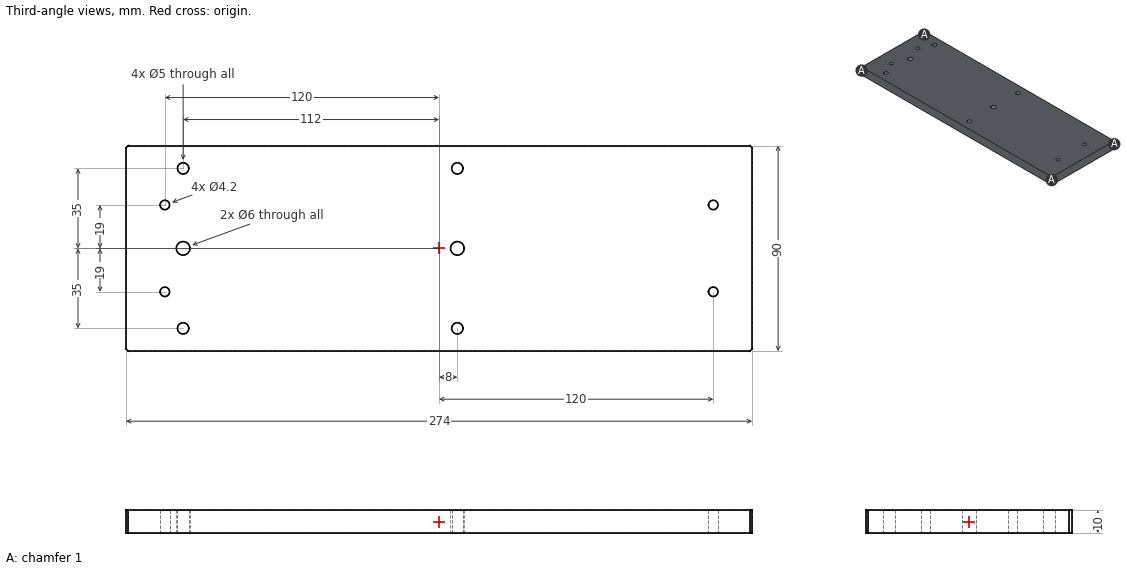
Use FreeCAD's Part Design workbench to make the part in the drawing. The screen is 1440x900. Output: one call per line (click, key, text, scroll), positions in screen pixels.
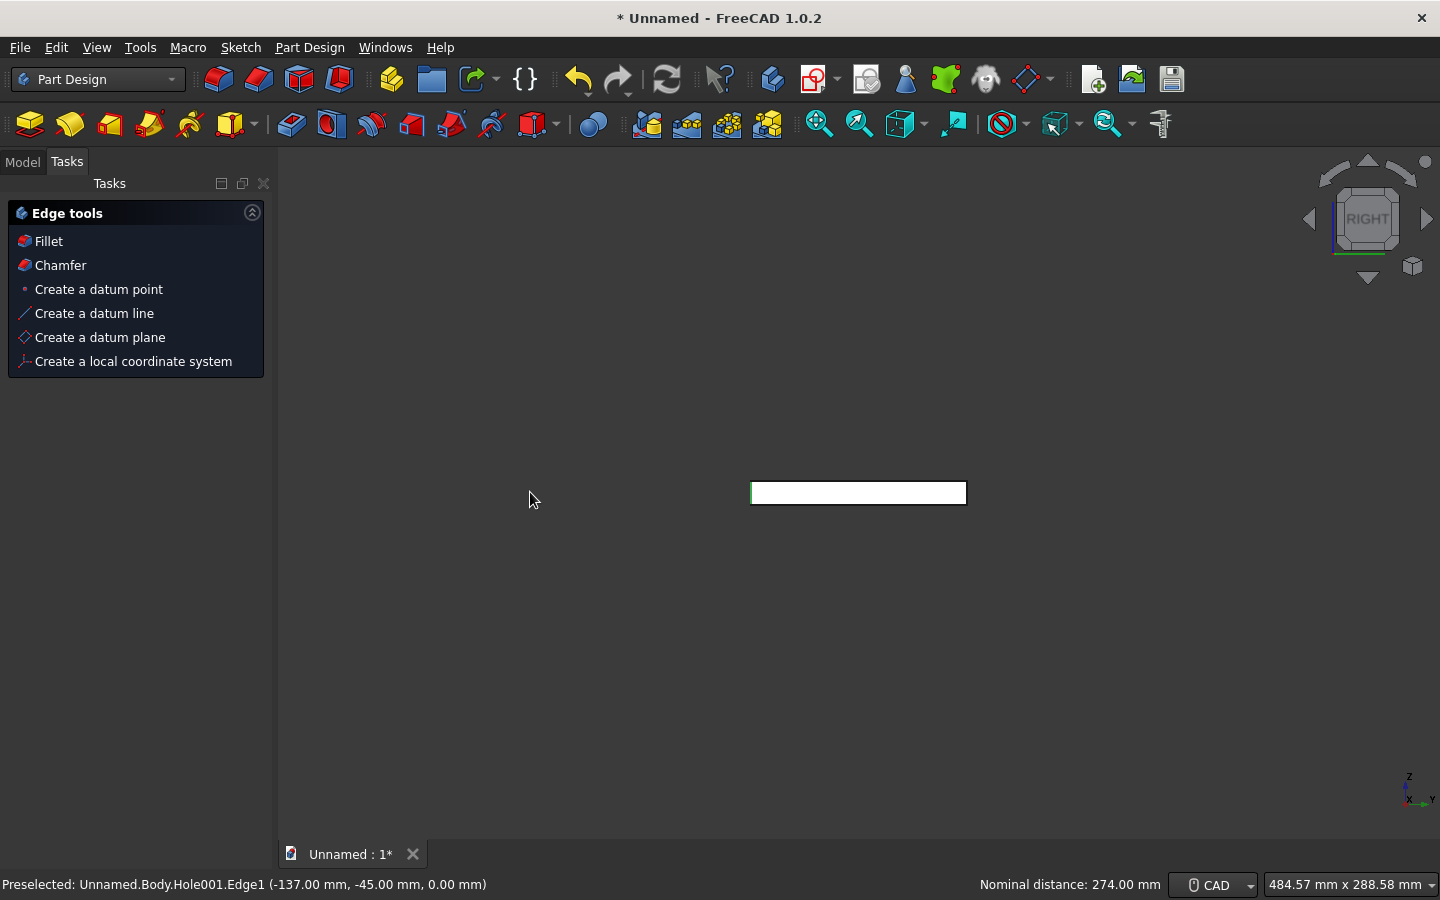
click(967, 492, ctrl)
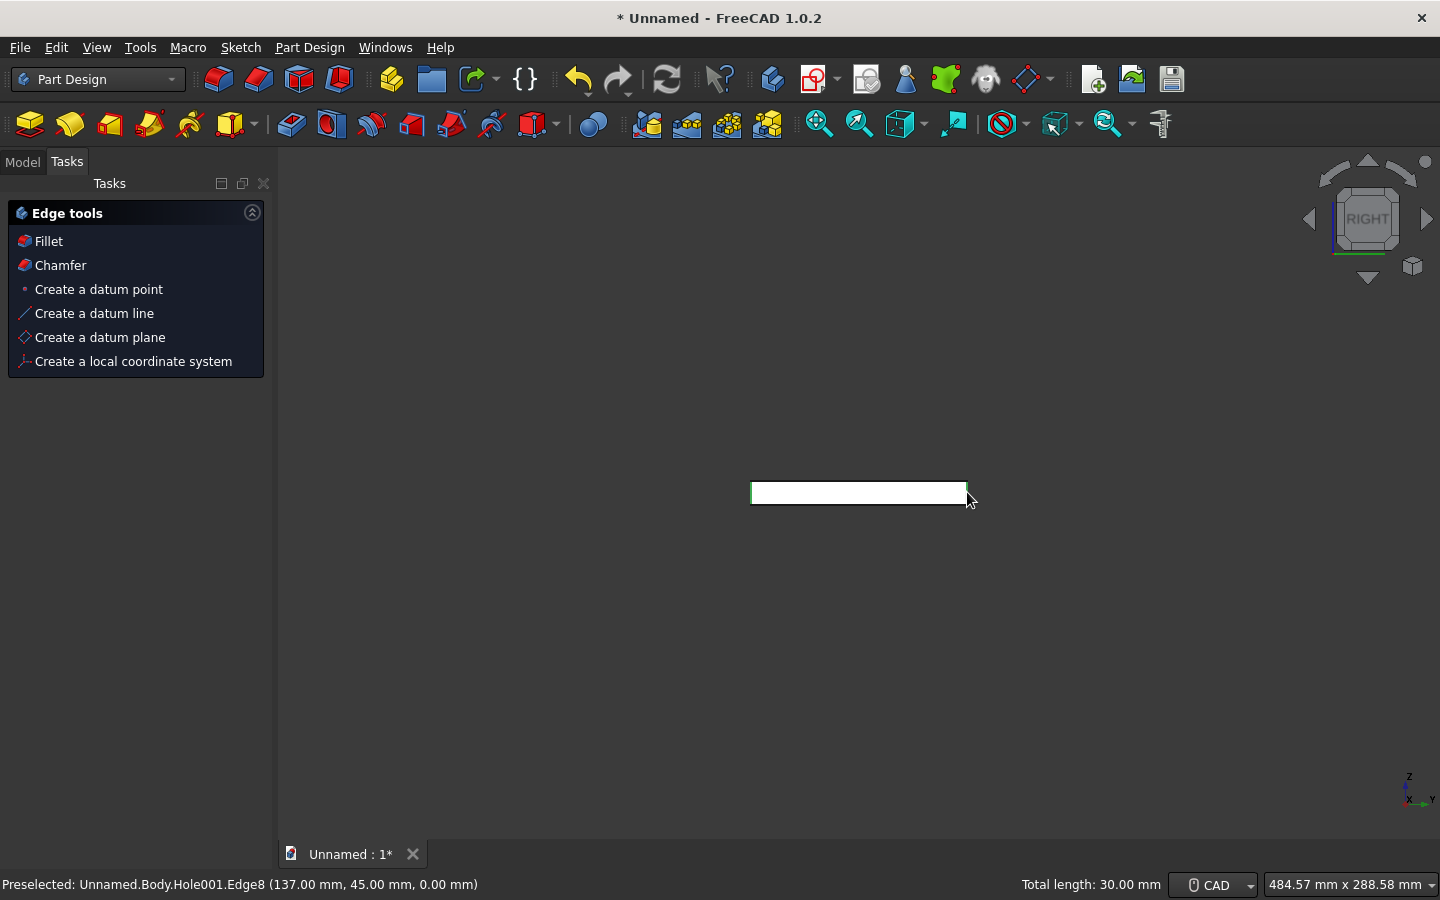
key(5)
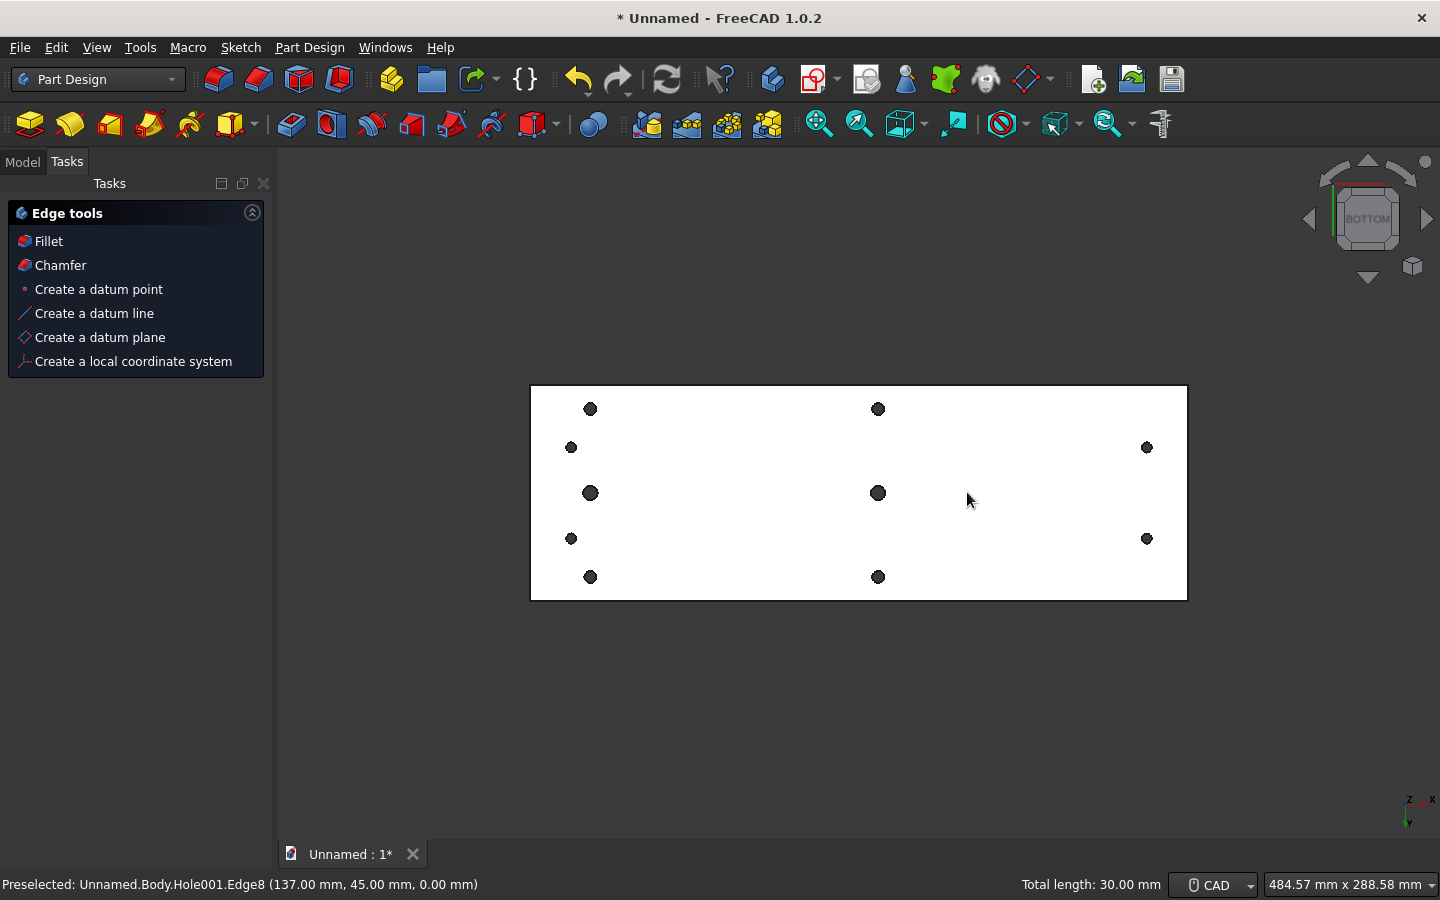
key(4)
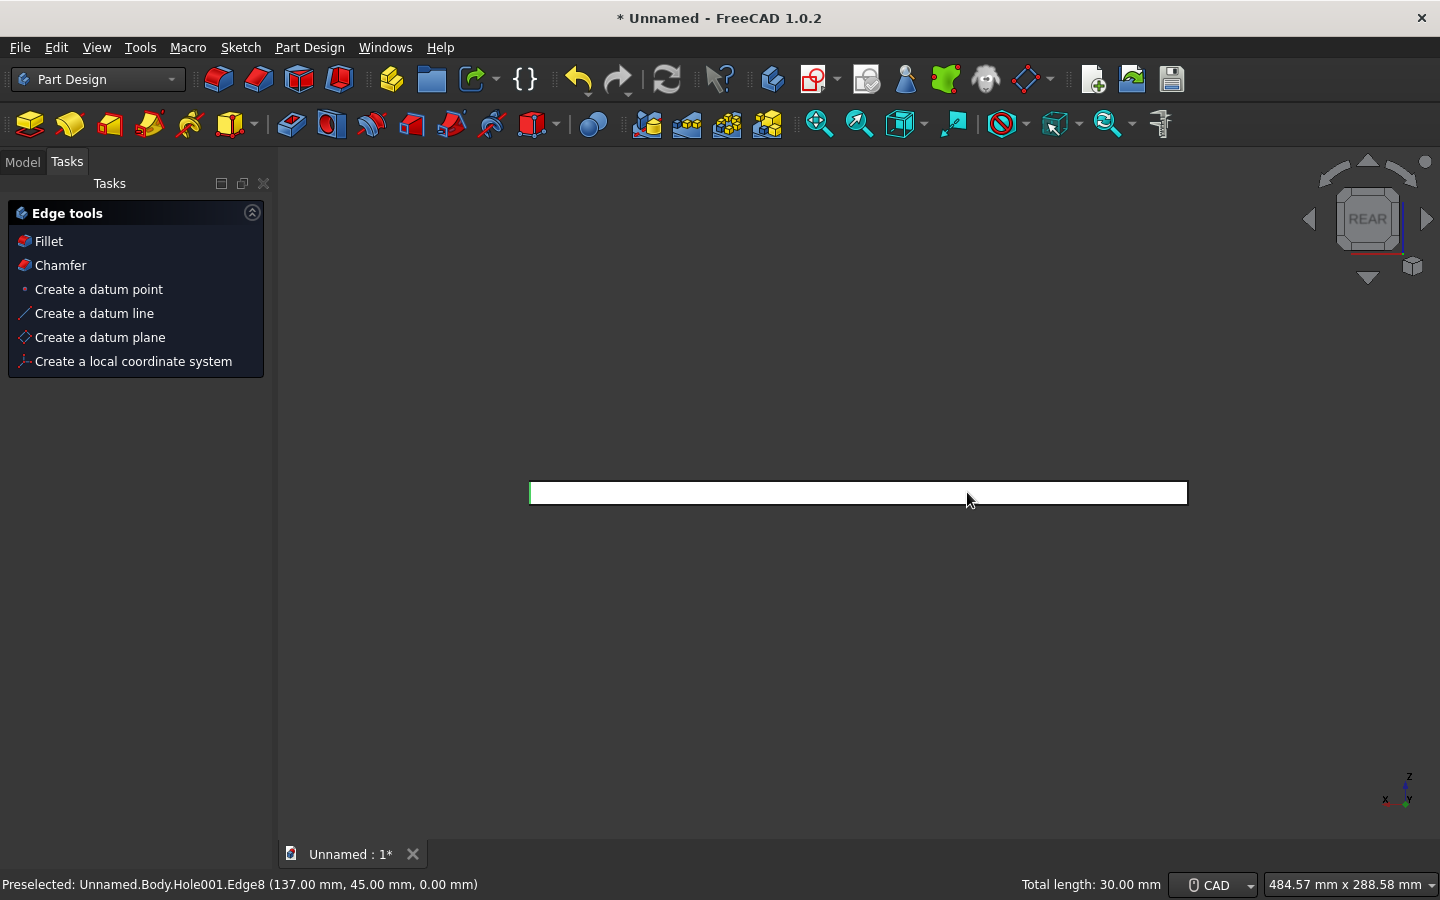
click(1188, 492, ctrl)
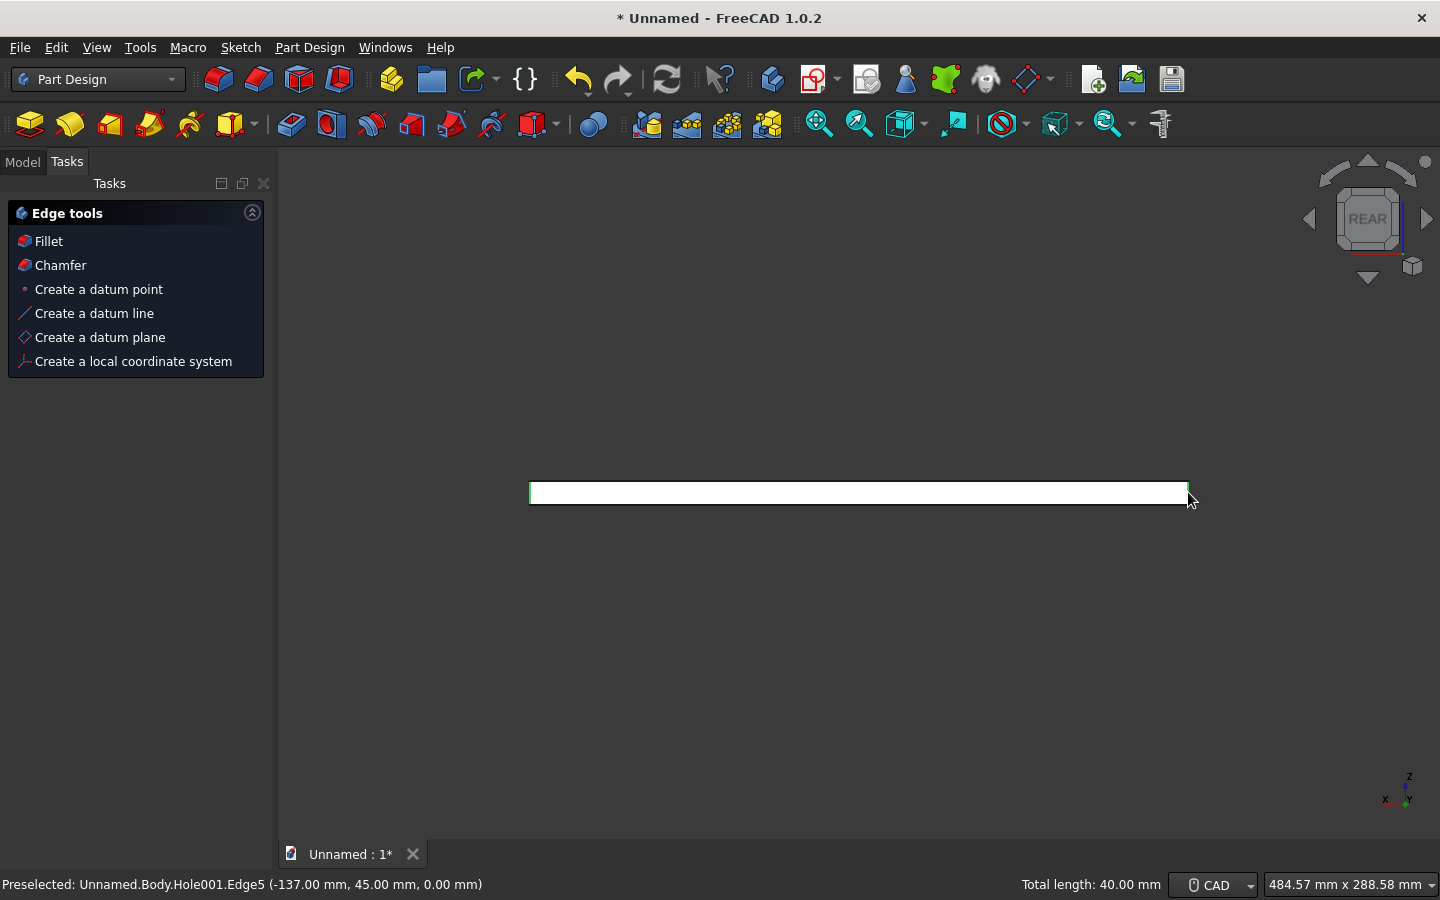
click(260, 80)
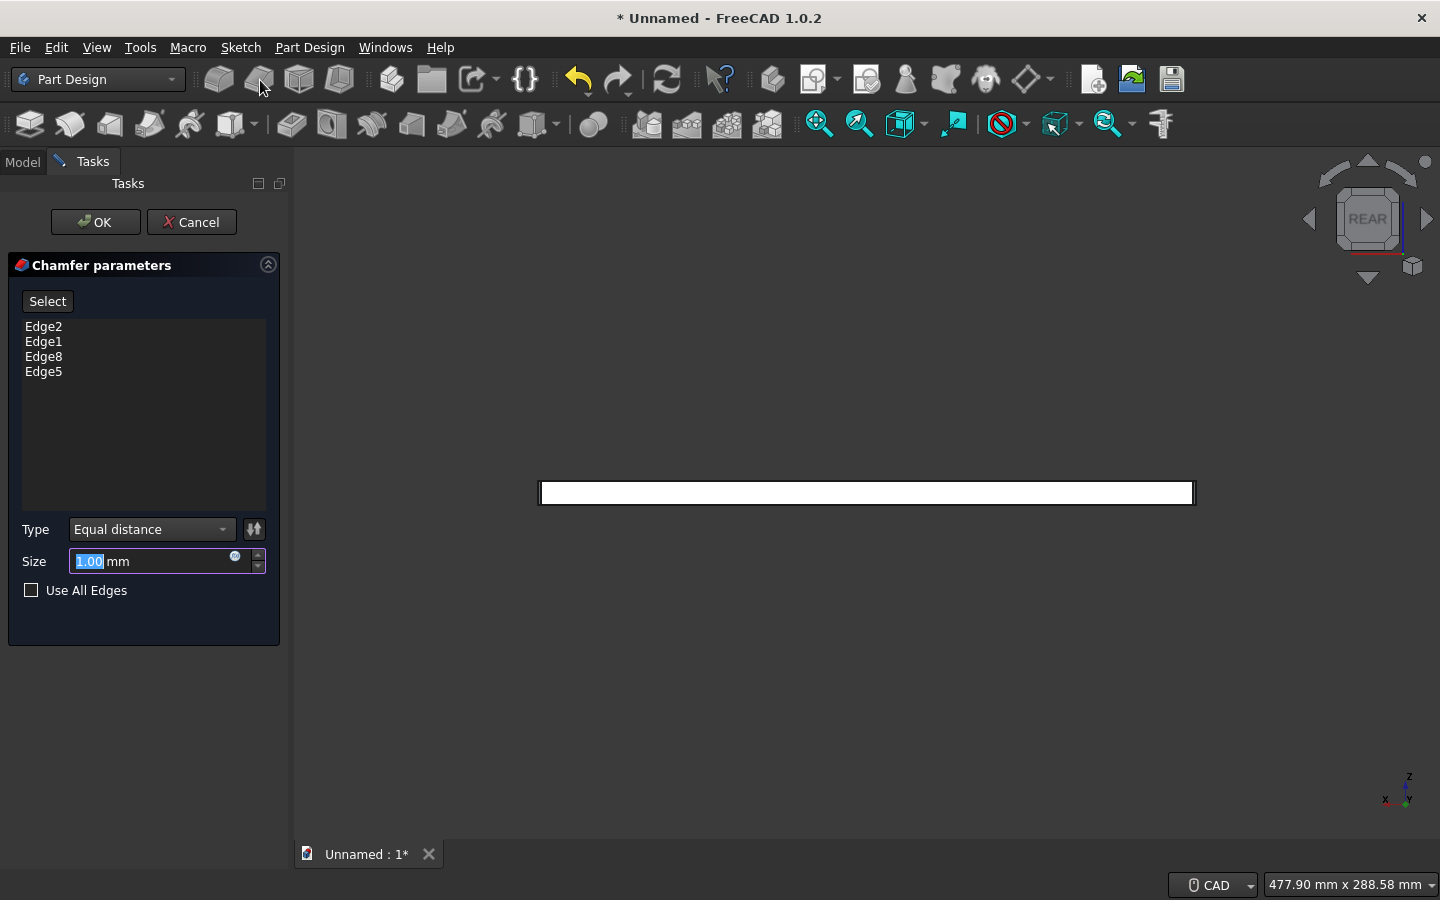
text(1)
key(Tab)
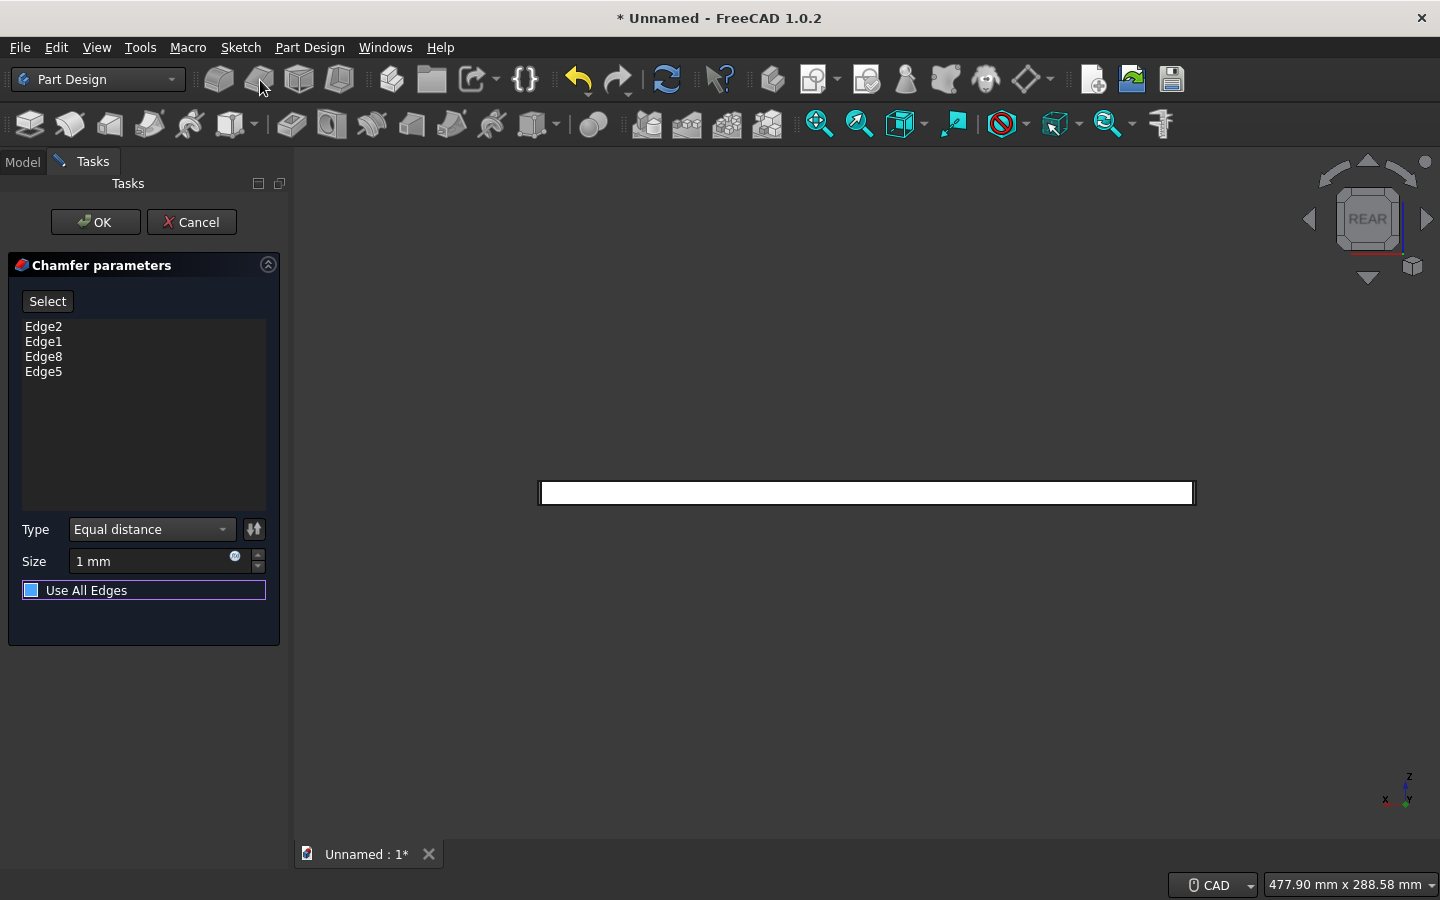
click(96, 222)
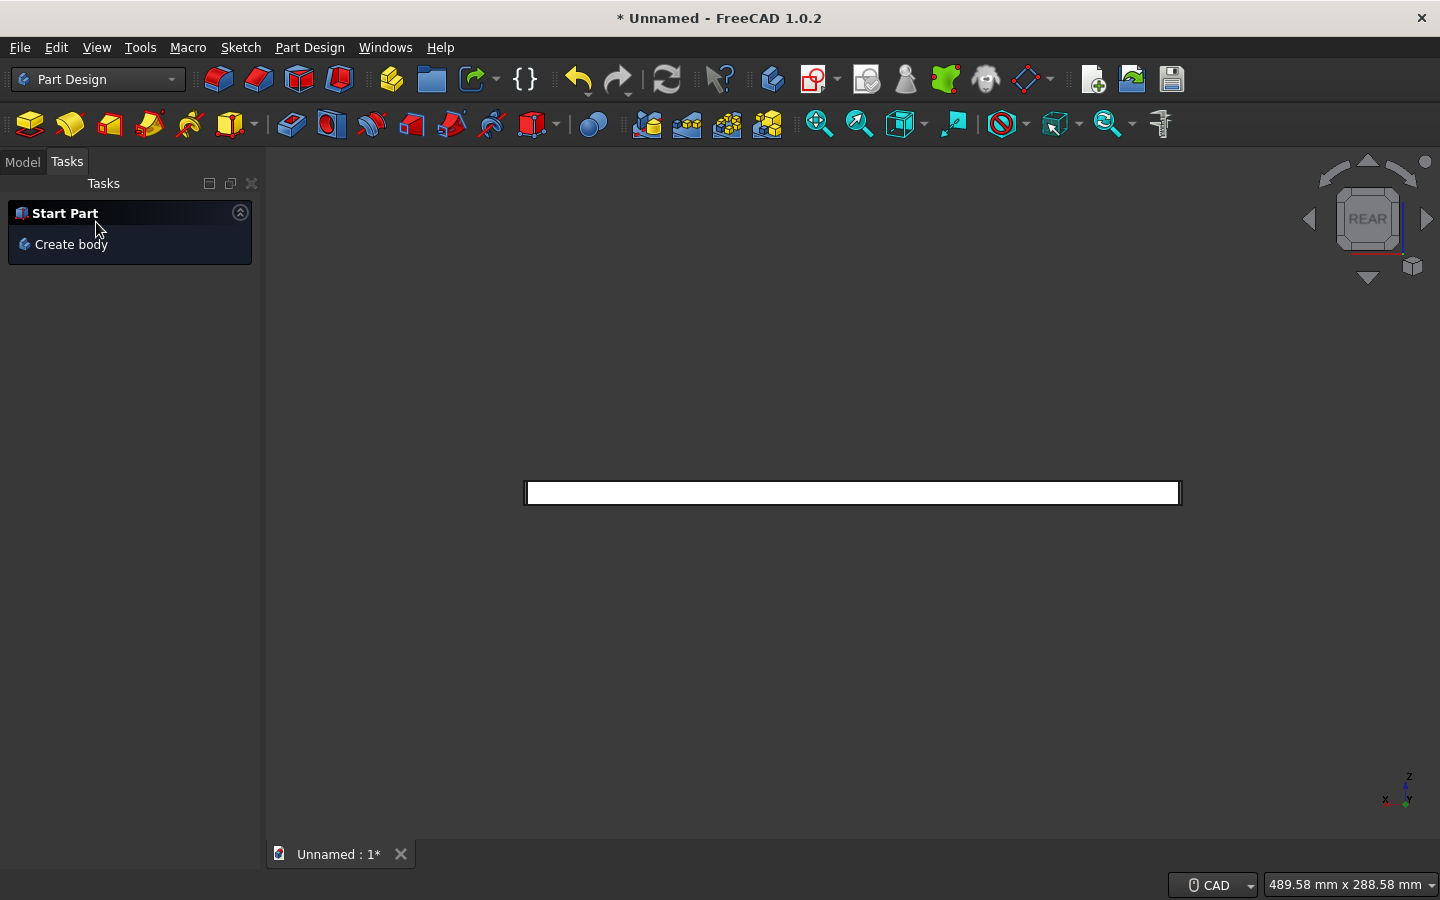
key(0)